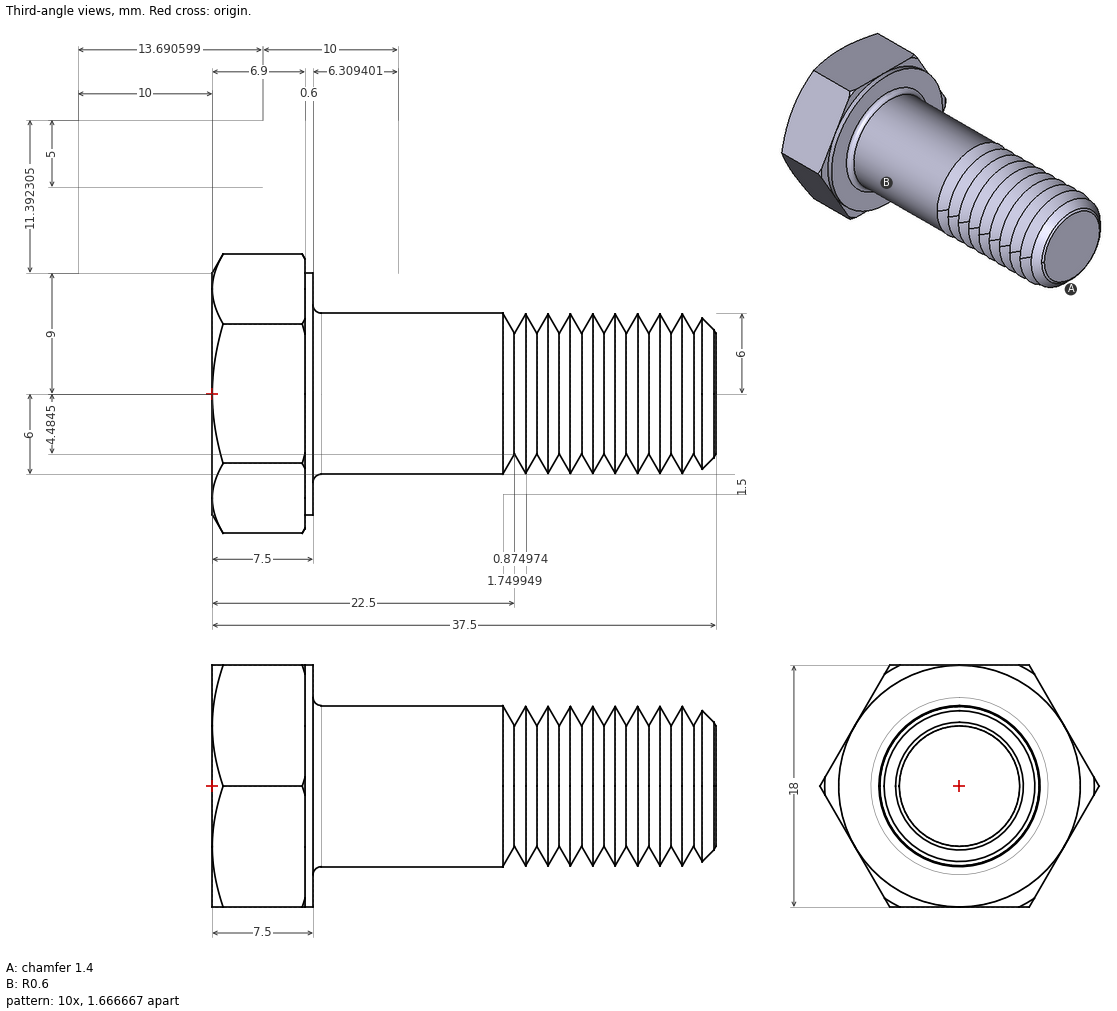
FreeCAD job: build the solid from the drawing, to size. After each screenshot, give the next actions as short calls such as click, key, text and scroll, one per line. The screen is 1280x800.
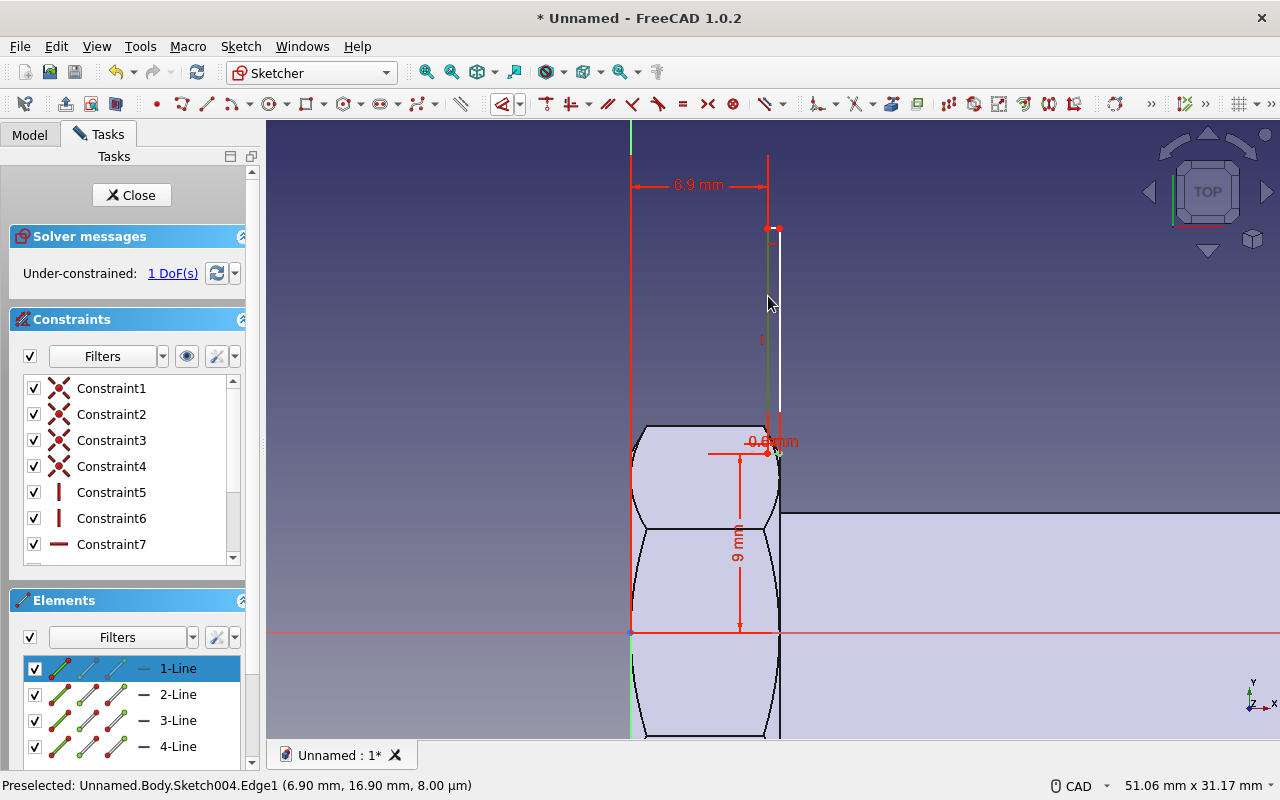
key(i)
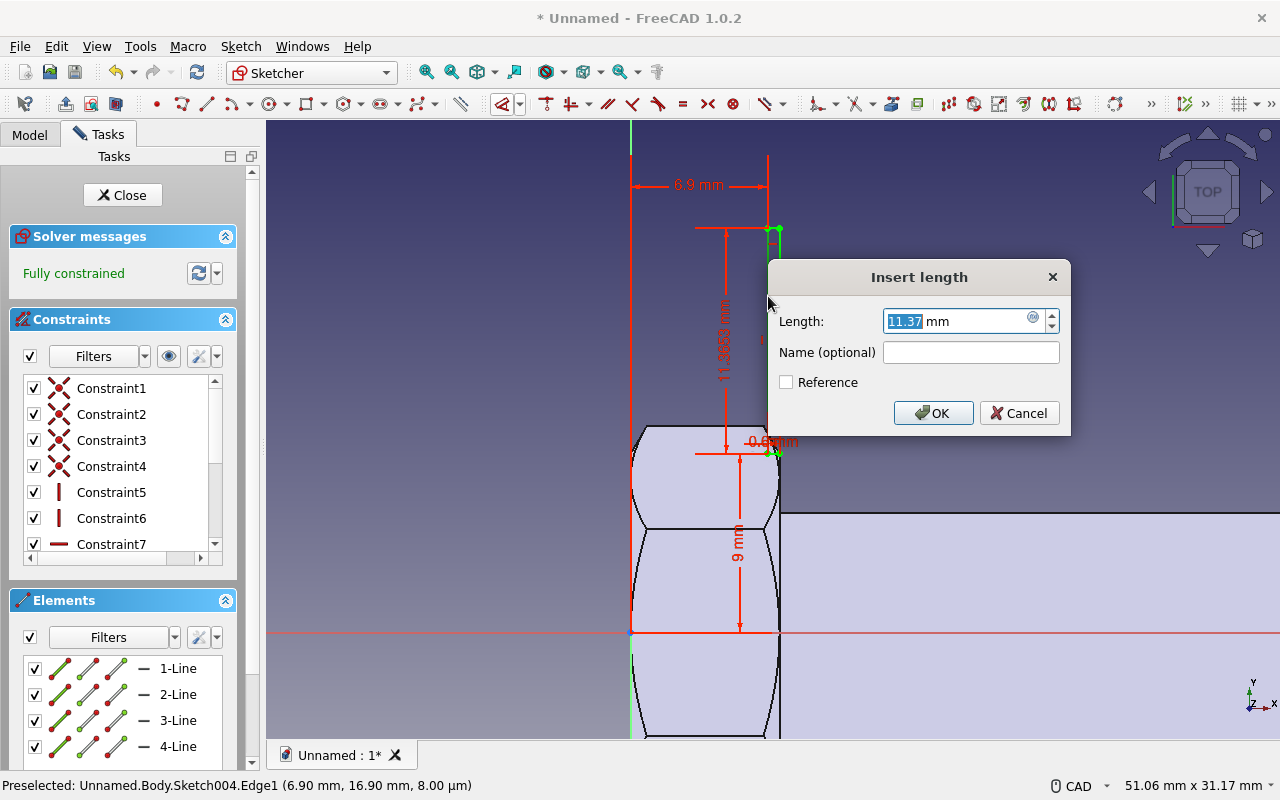
text(11.392305)
key(Return)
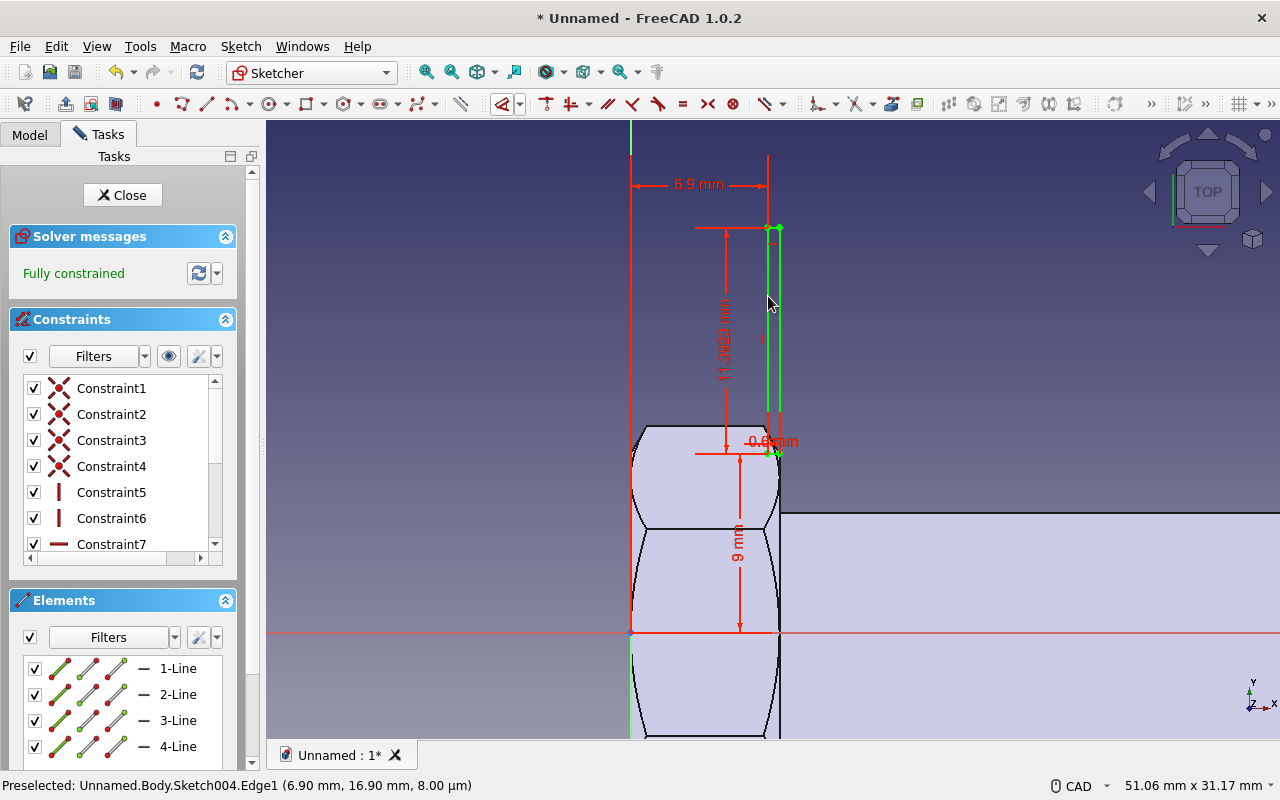
click(123, 195)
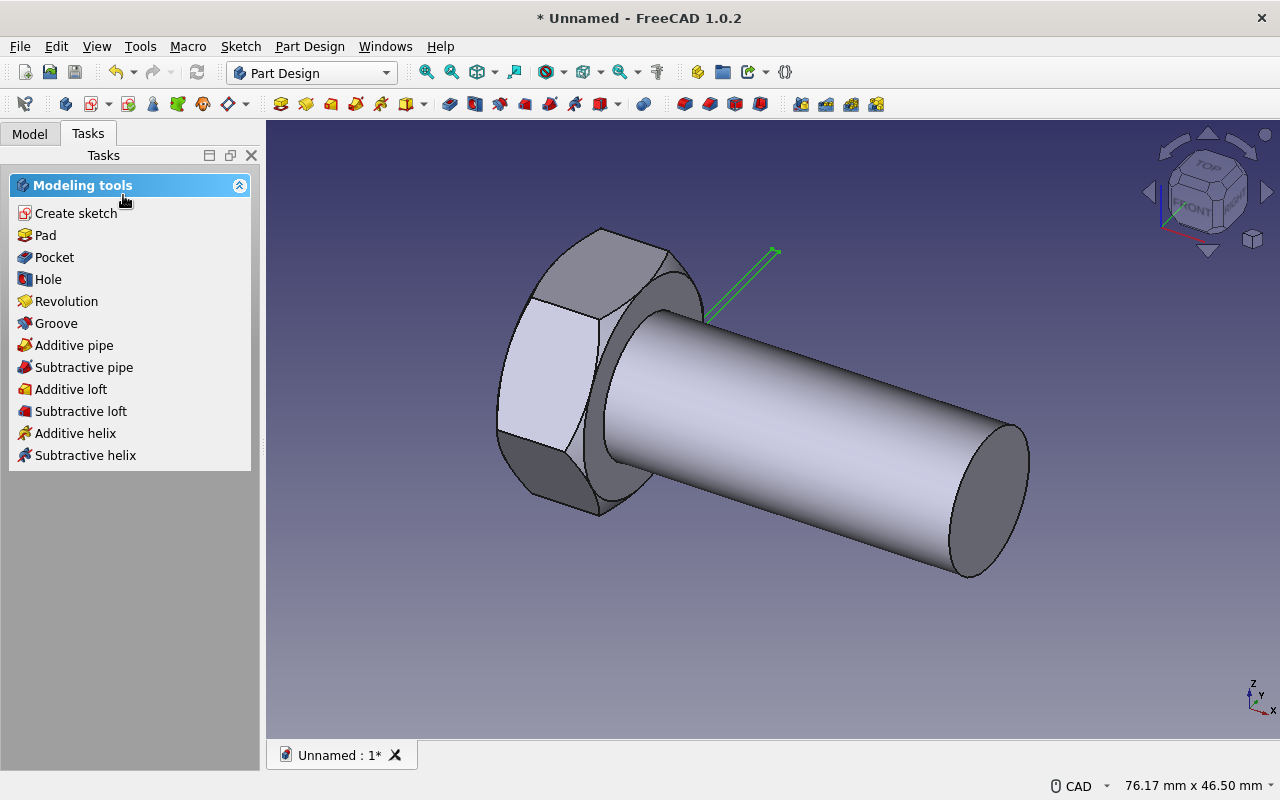
click(500, 104)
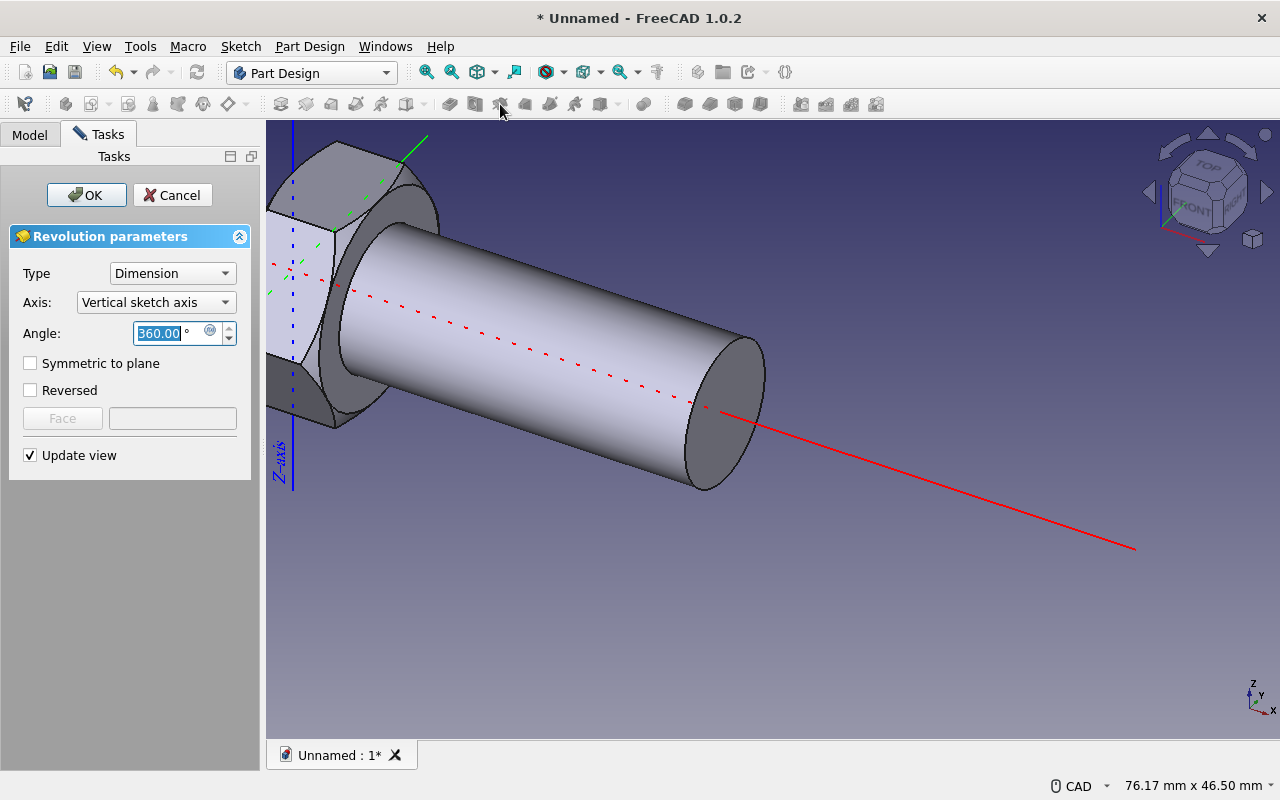
click(157, 302)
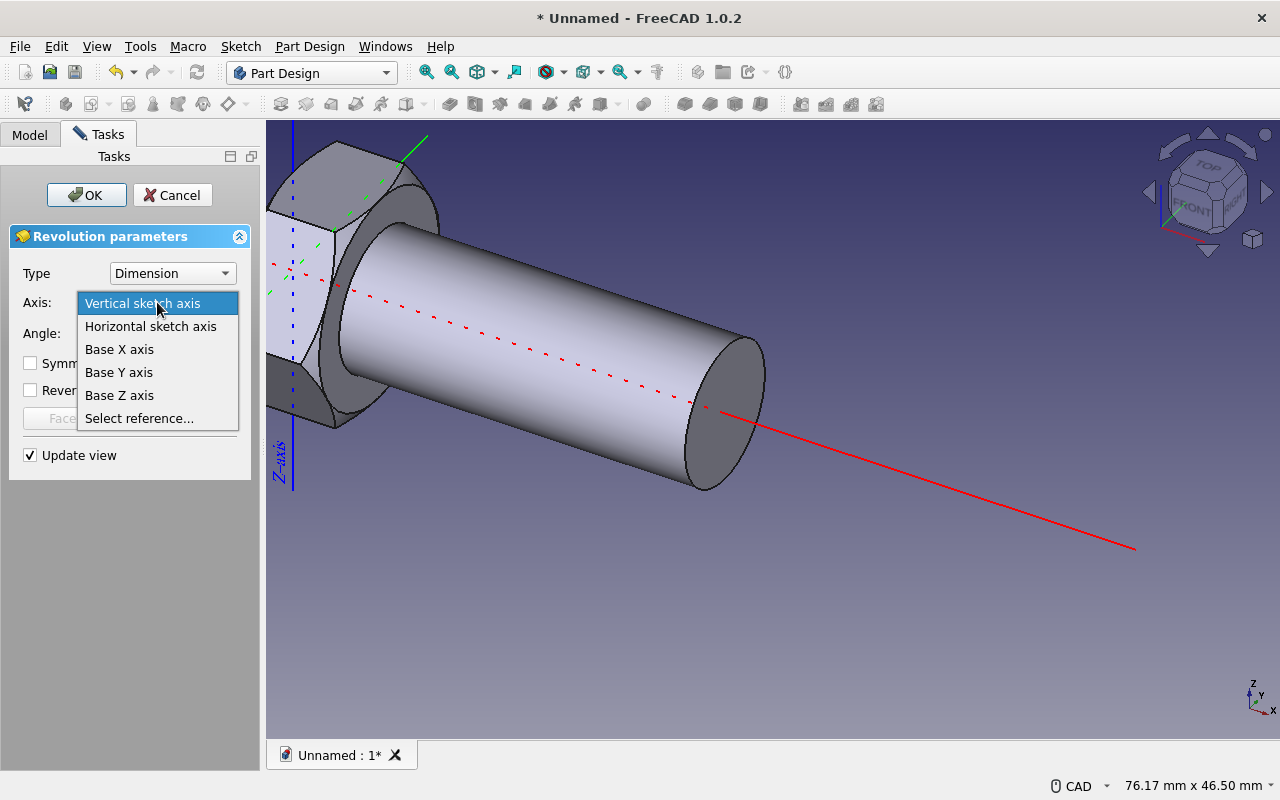
click(156, 326)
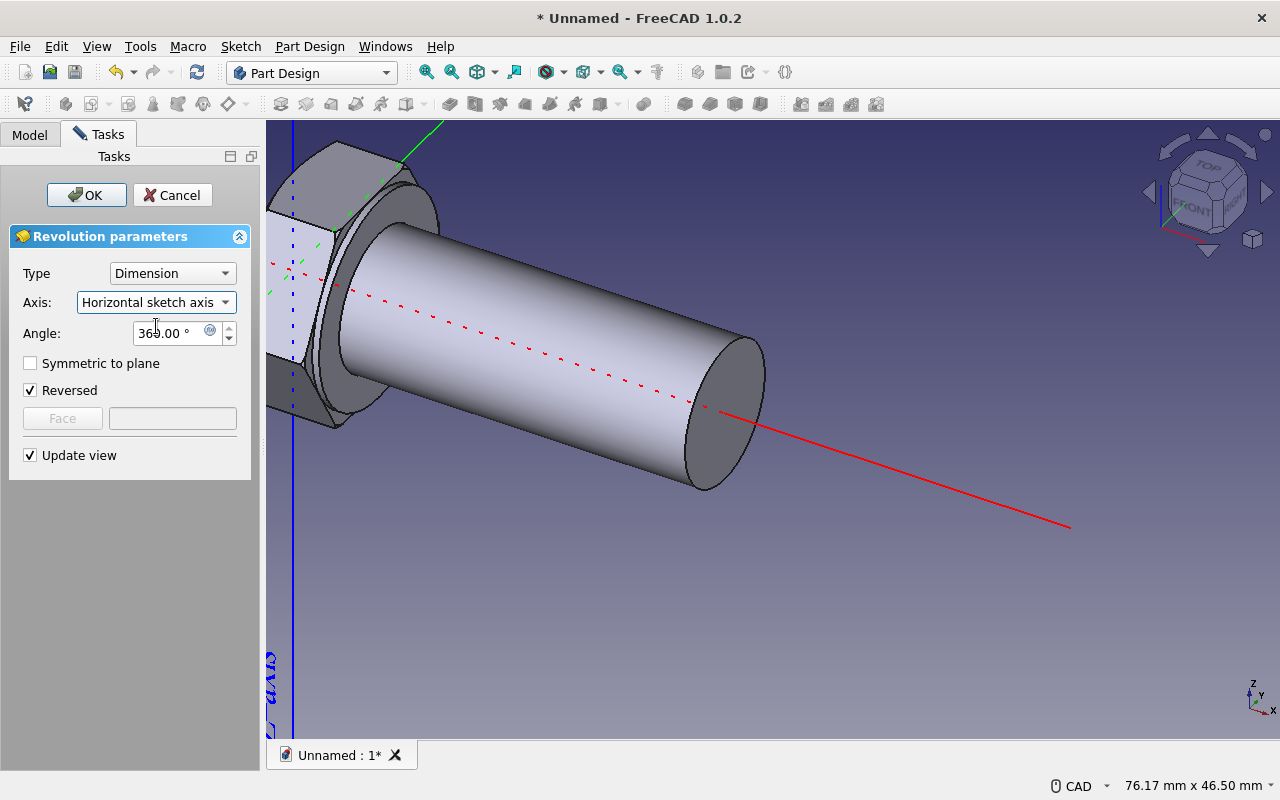
click(87, 195)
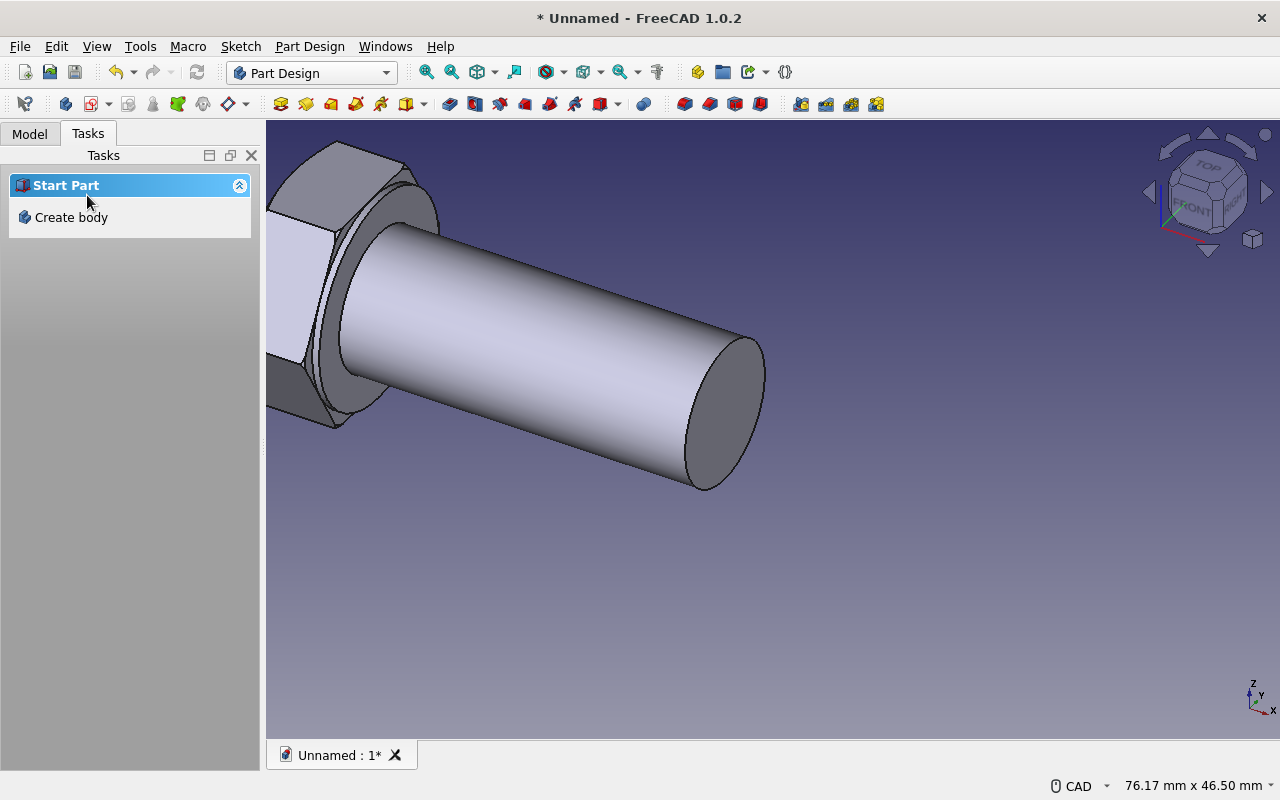
click(427, 72)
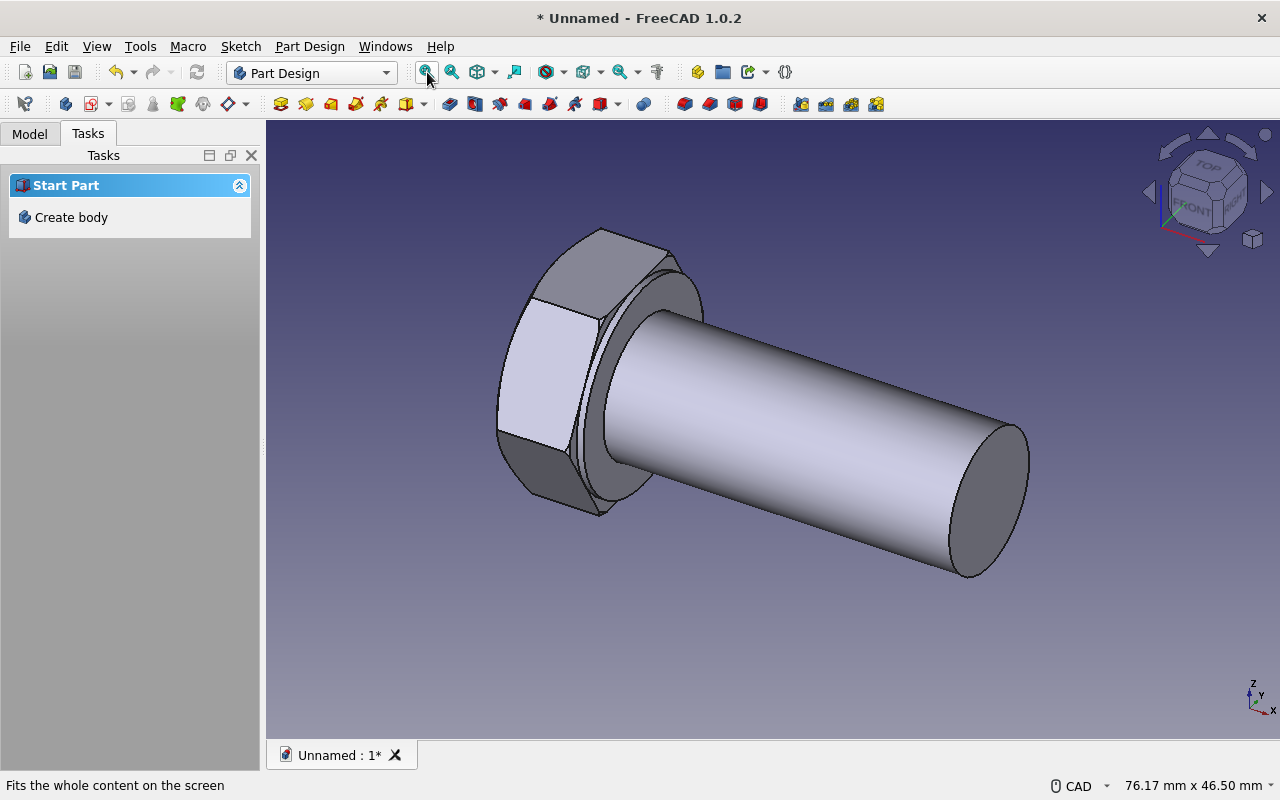
click(949, 540)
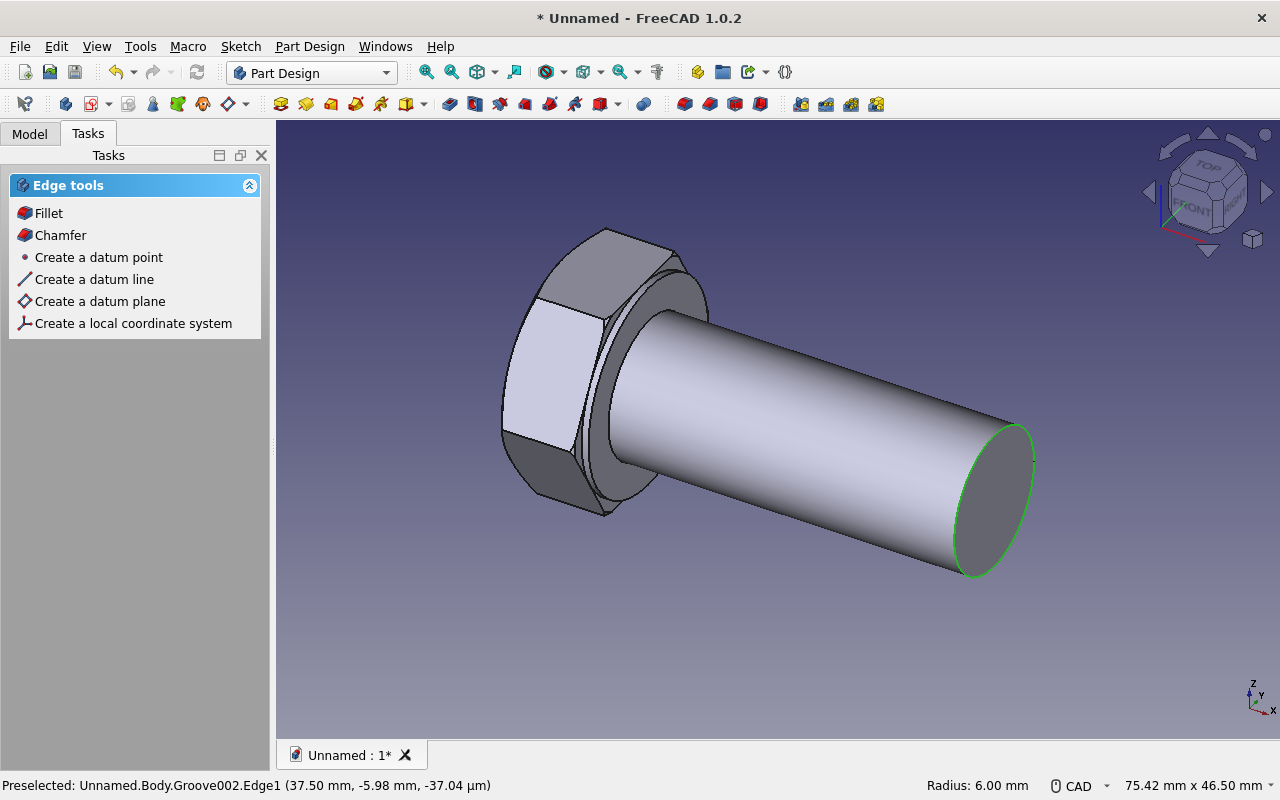
click(710, 104)